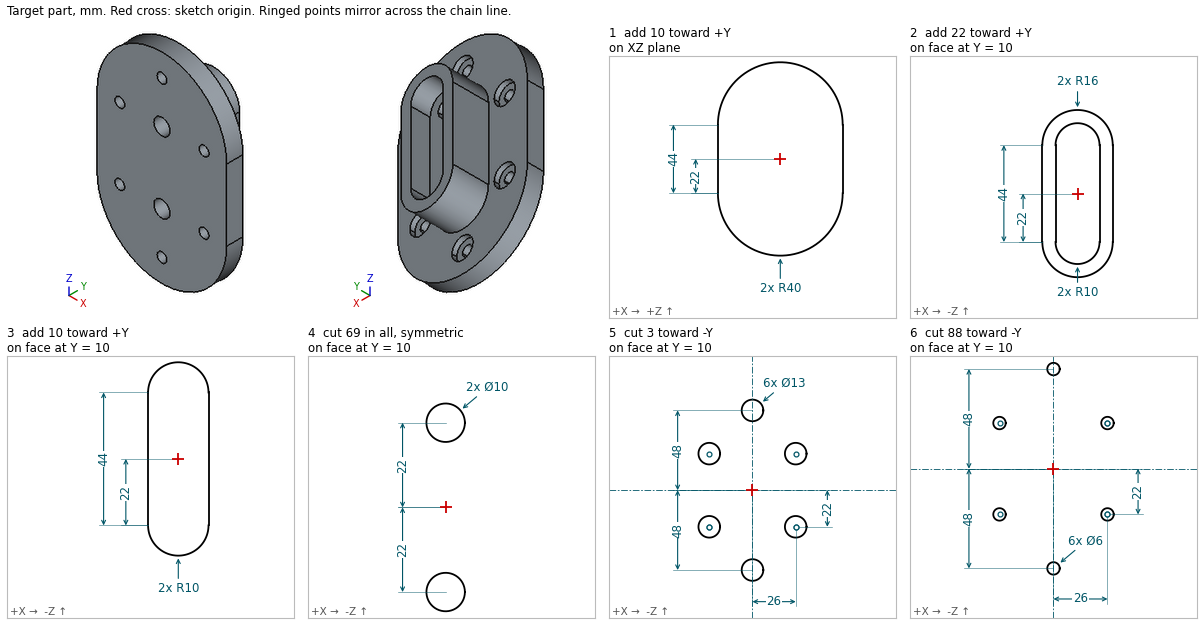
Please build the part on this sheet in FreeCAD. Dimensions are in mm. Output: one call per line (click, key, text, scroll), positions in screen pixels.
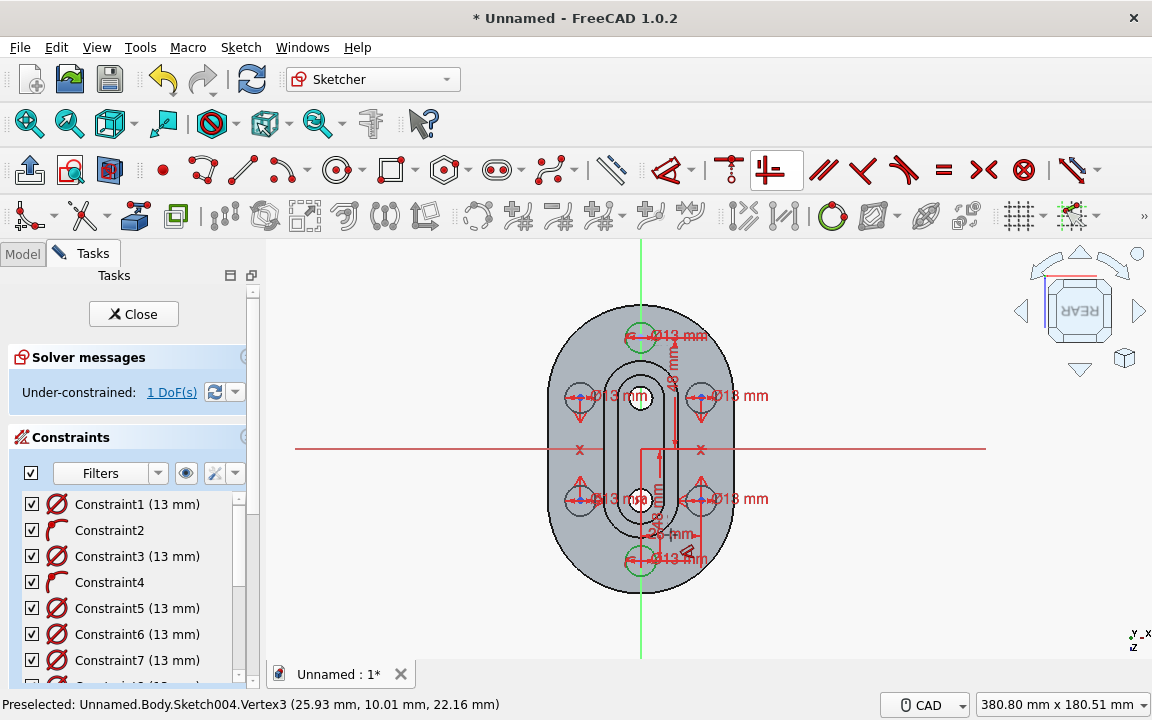
click(701, 501)
click(735, 475)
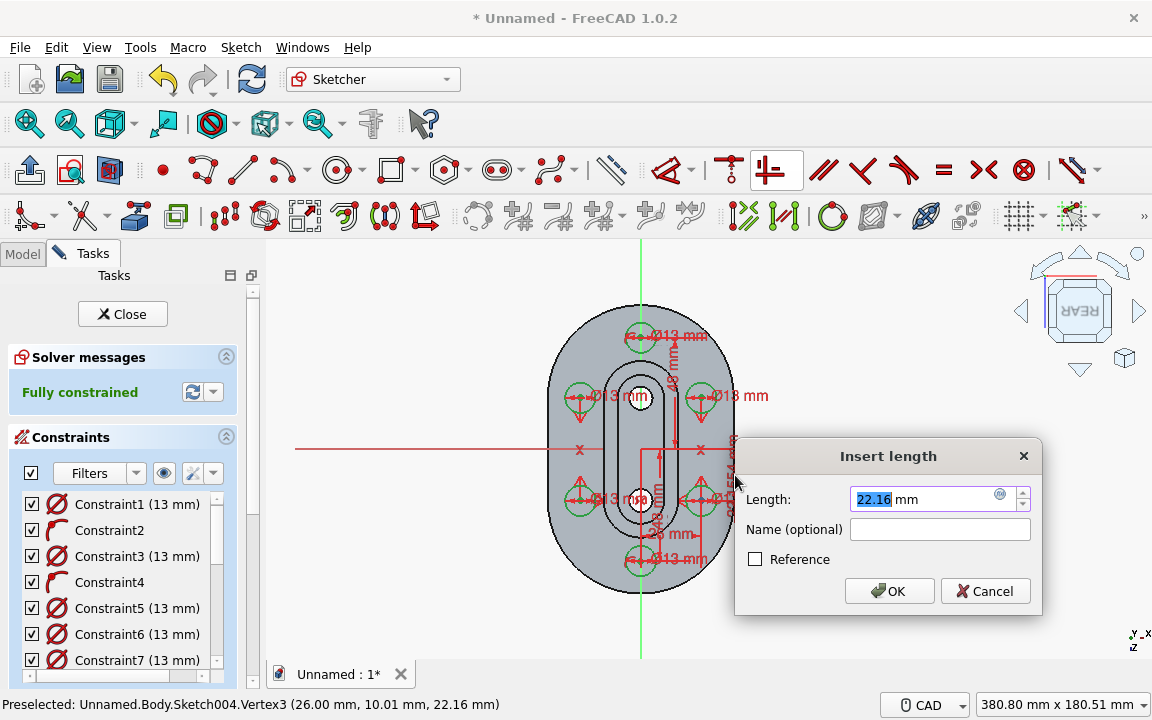
text(22)
key(Return)
key(Escape)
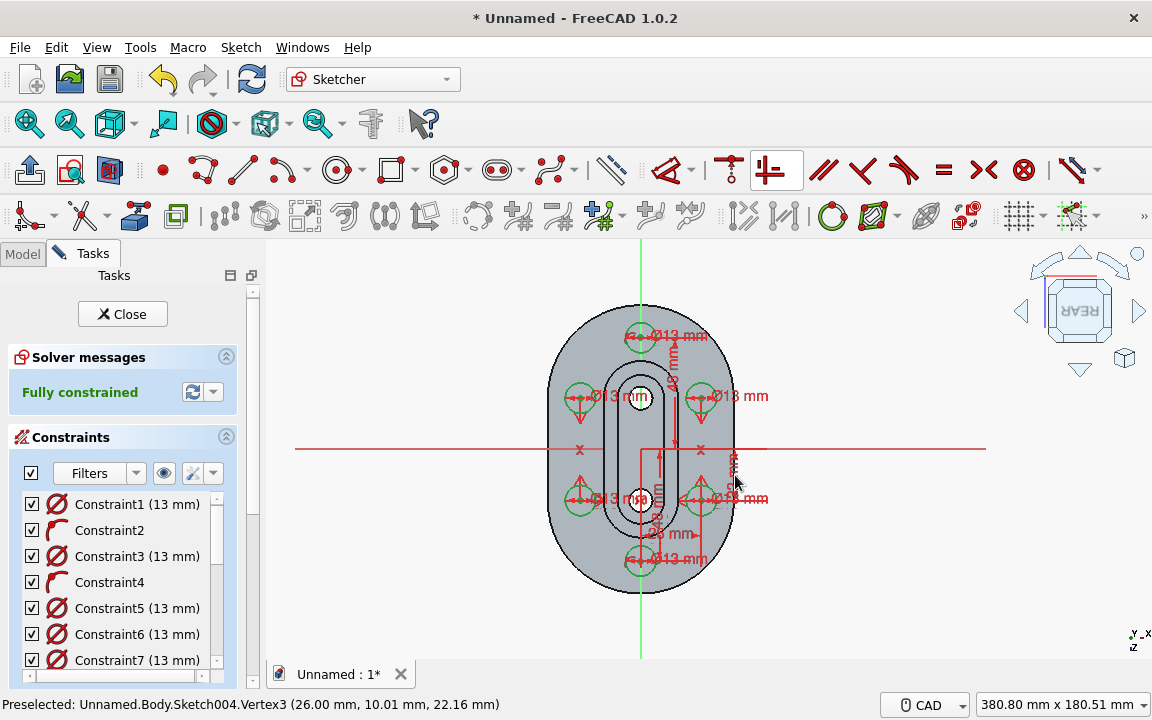
click(123, 314)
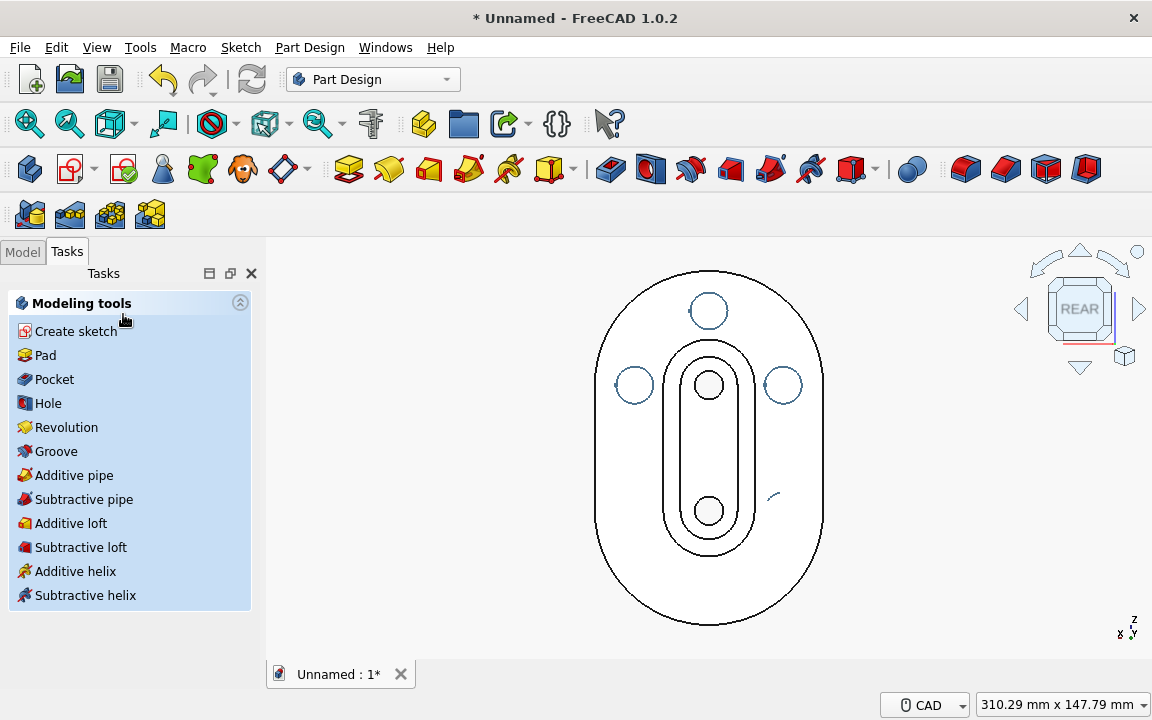
click(612, 170)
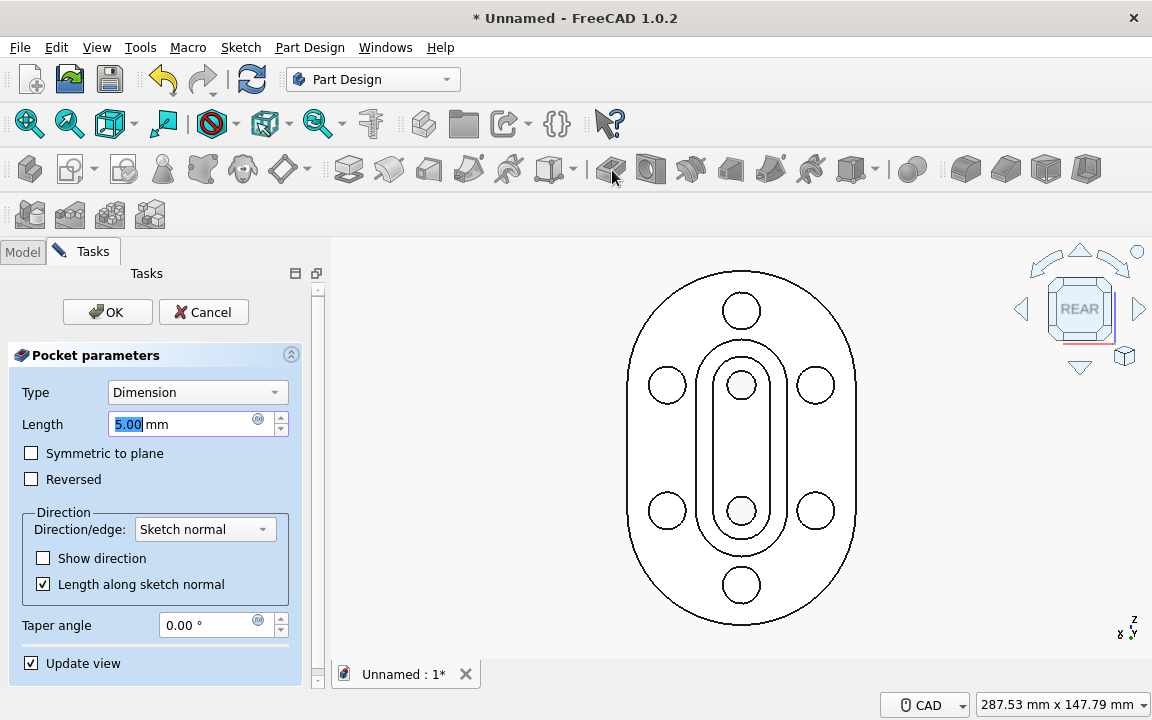
text(3)
key(Tab)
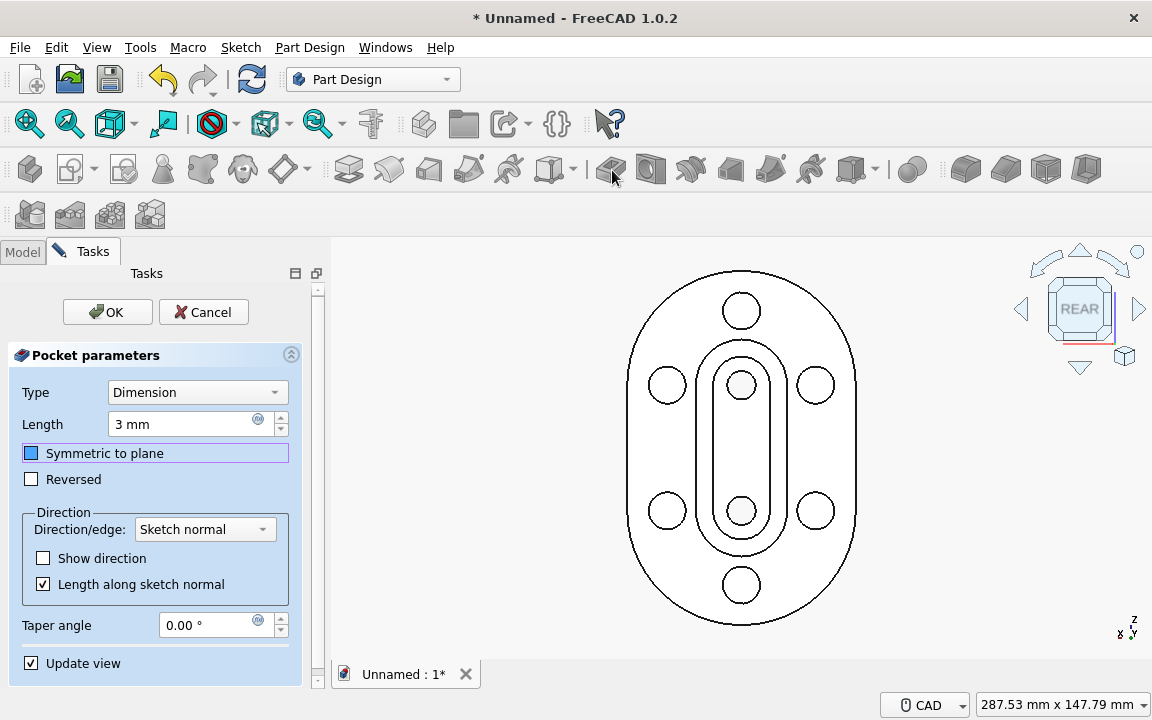
click(108, 312)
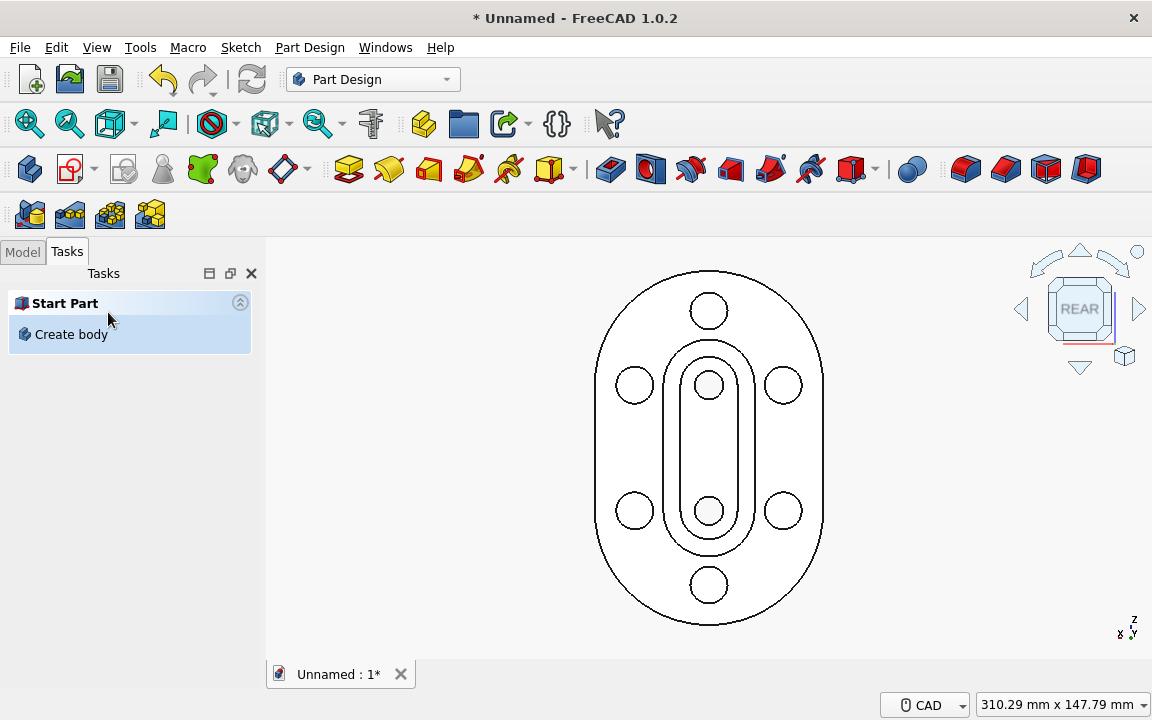
click(644, 346)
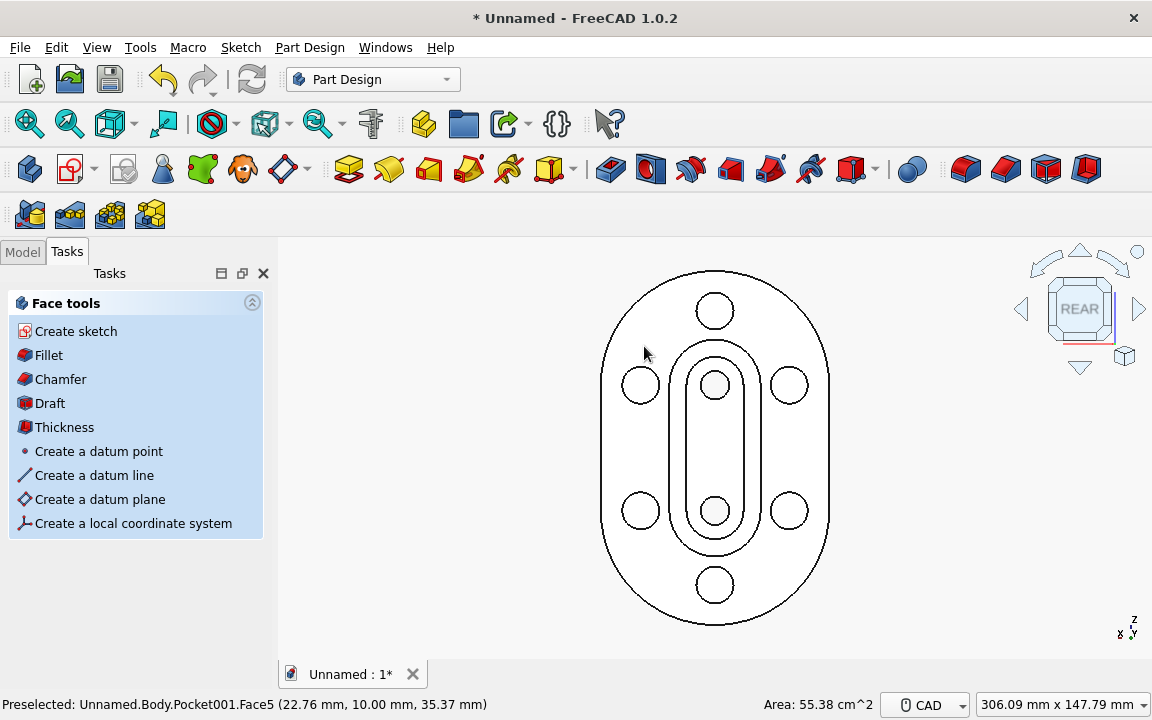
click(70, 170)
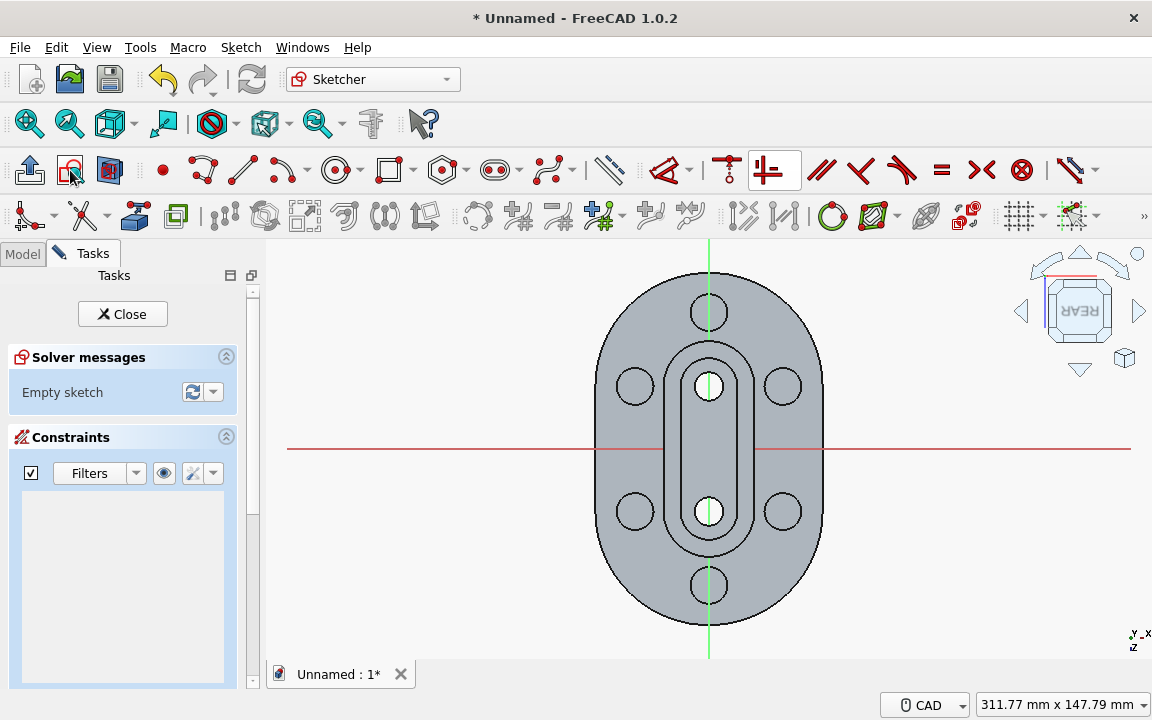
click(110, 170)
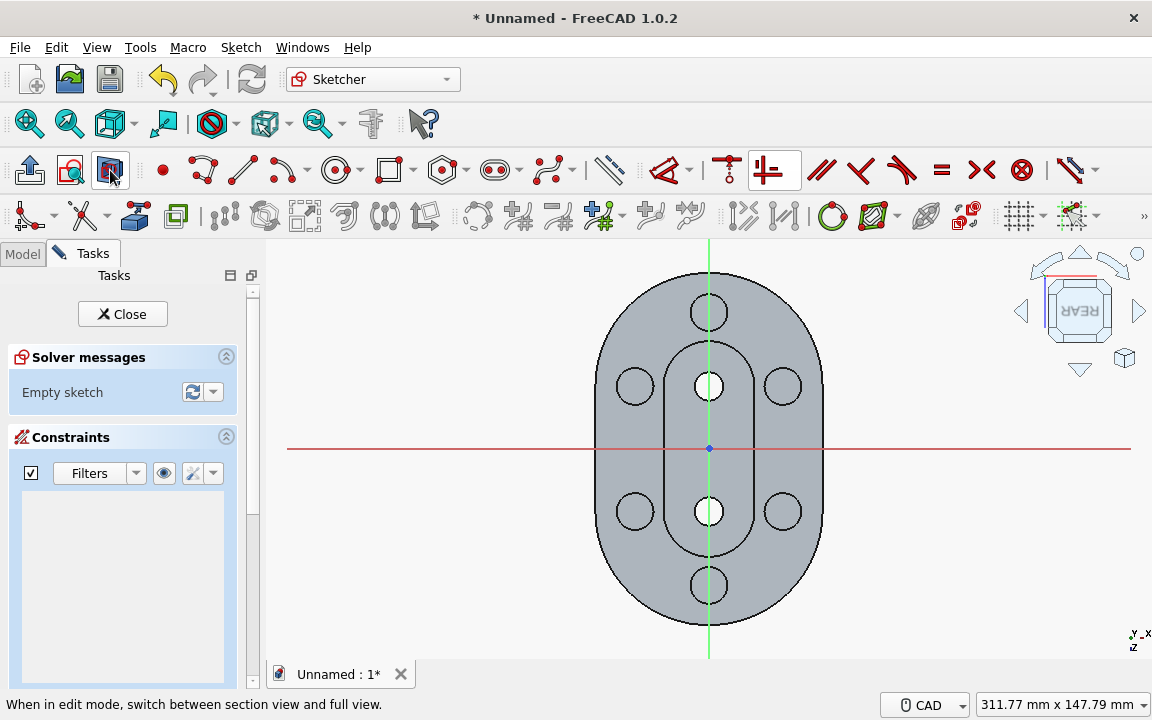
click(336, 170)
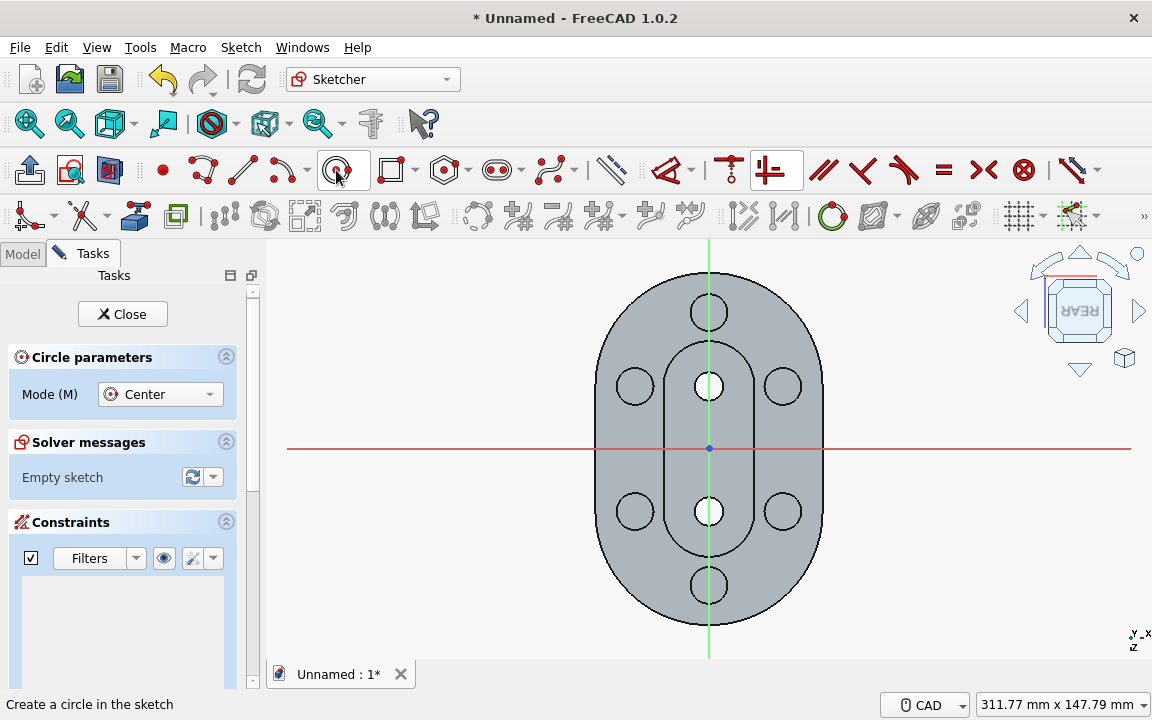
scroll(709, 585, up, 5)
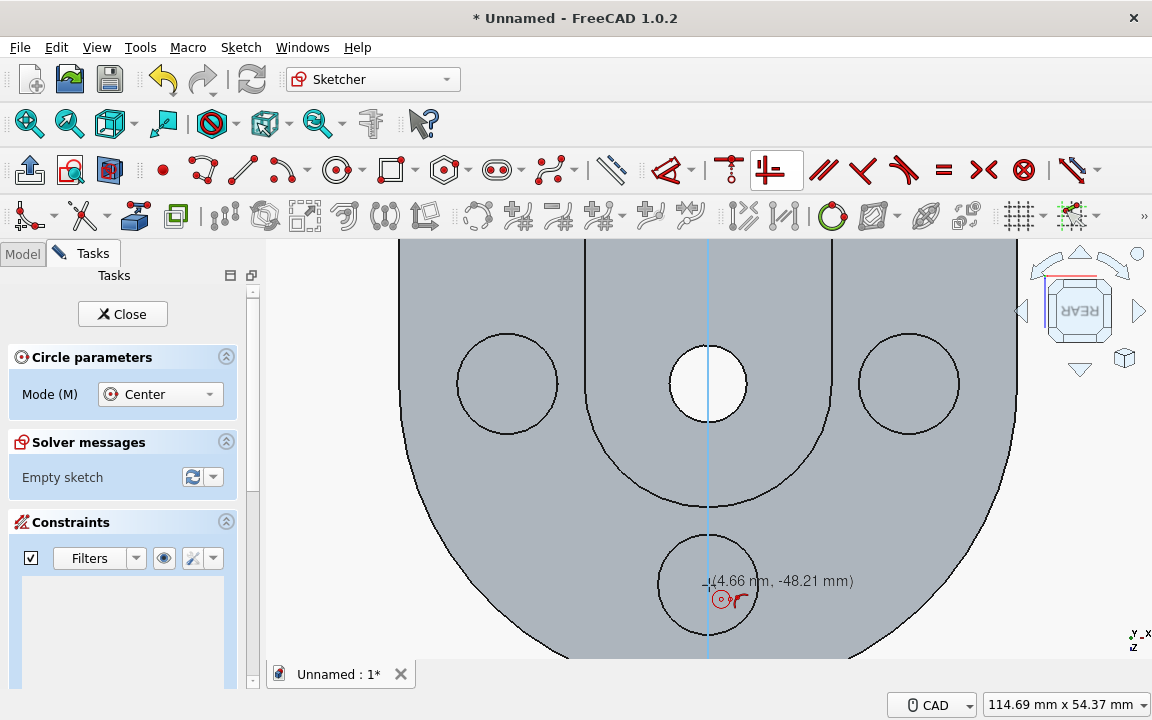
click(708, 585)
move(725, 568)